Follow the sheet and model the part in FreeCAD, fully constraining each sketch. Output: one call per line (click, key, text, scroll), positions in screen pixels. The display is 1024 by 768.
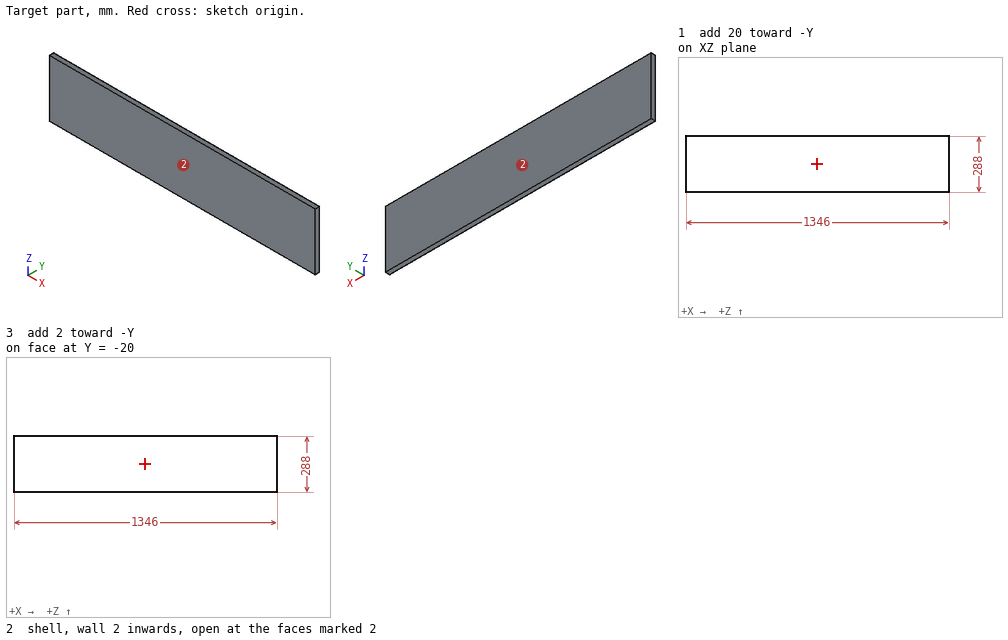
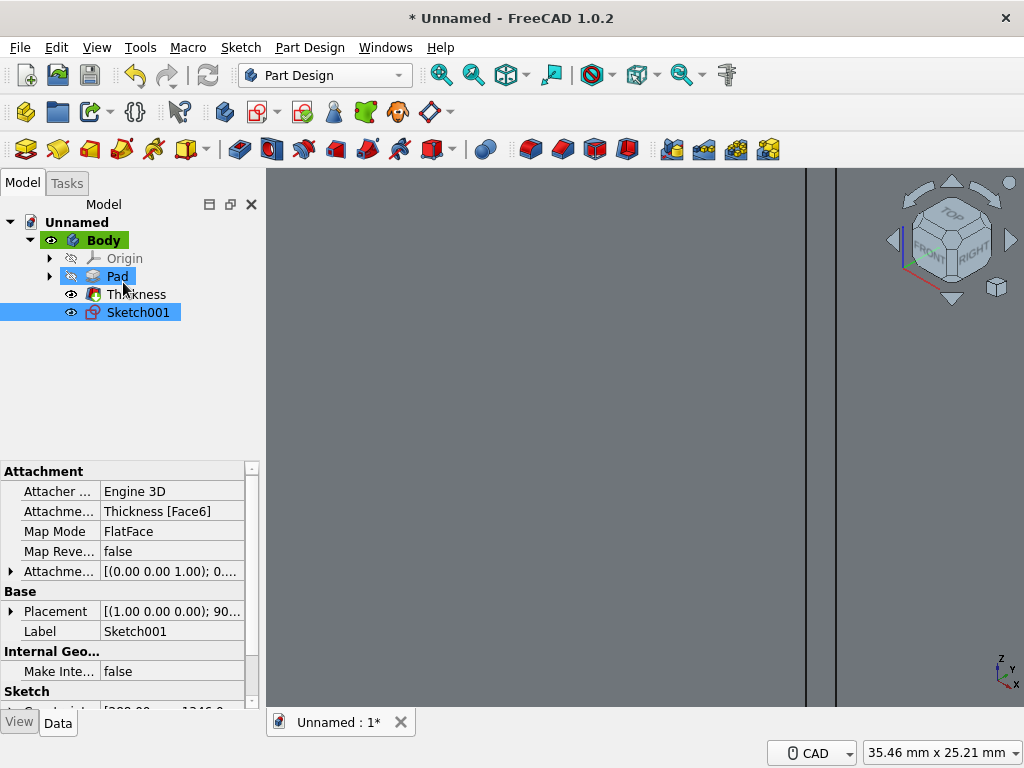
click(26, 150)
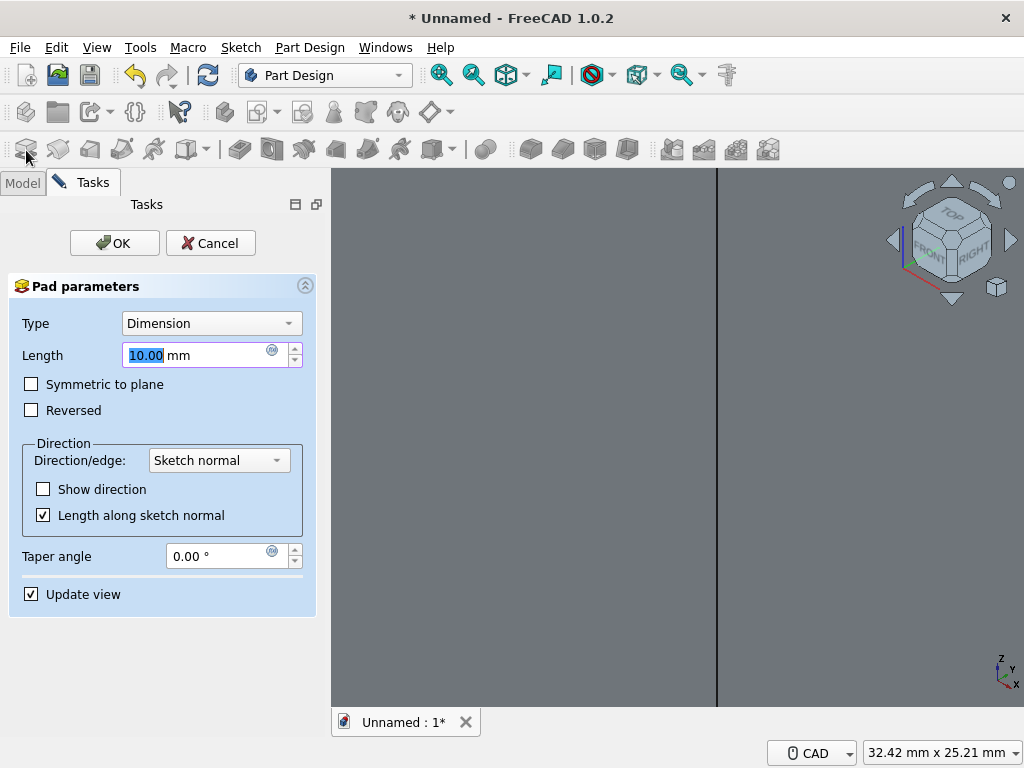
text(2)
key(Tab)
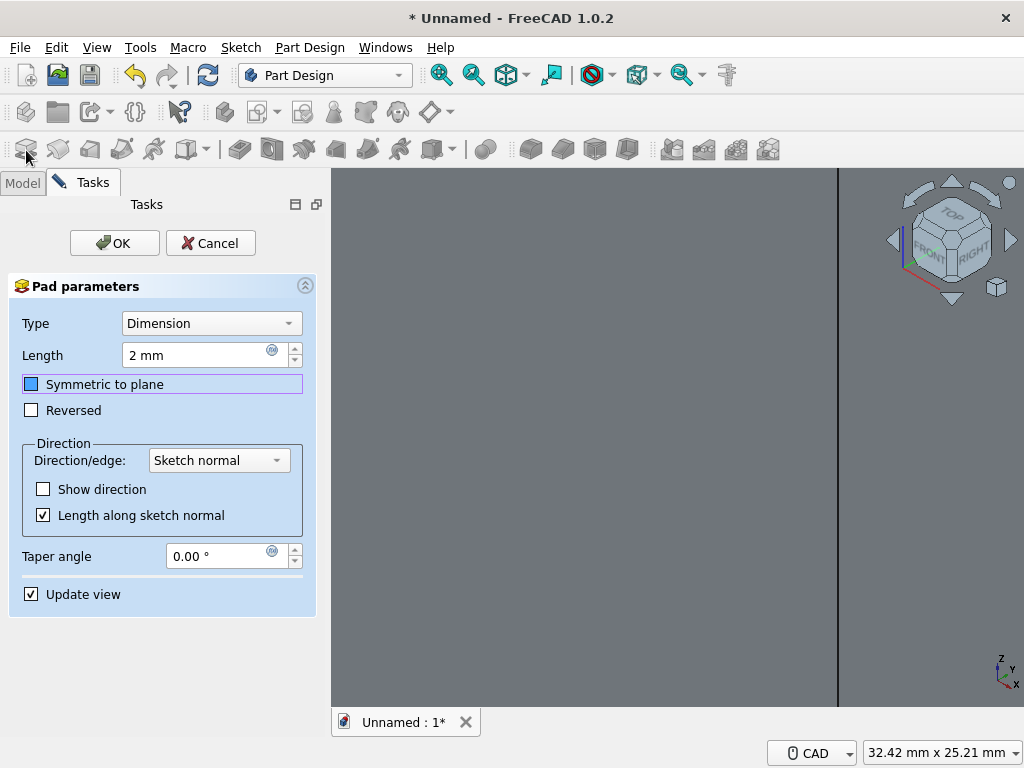
click(115, 243)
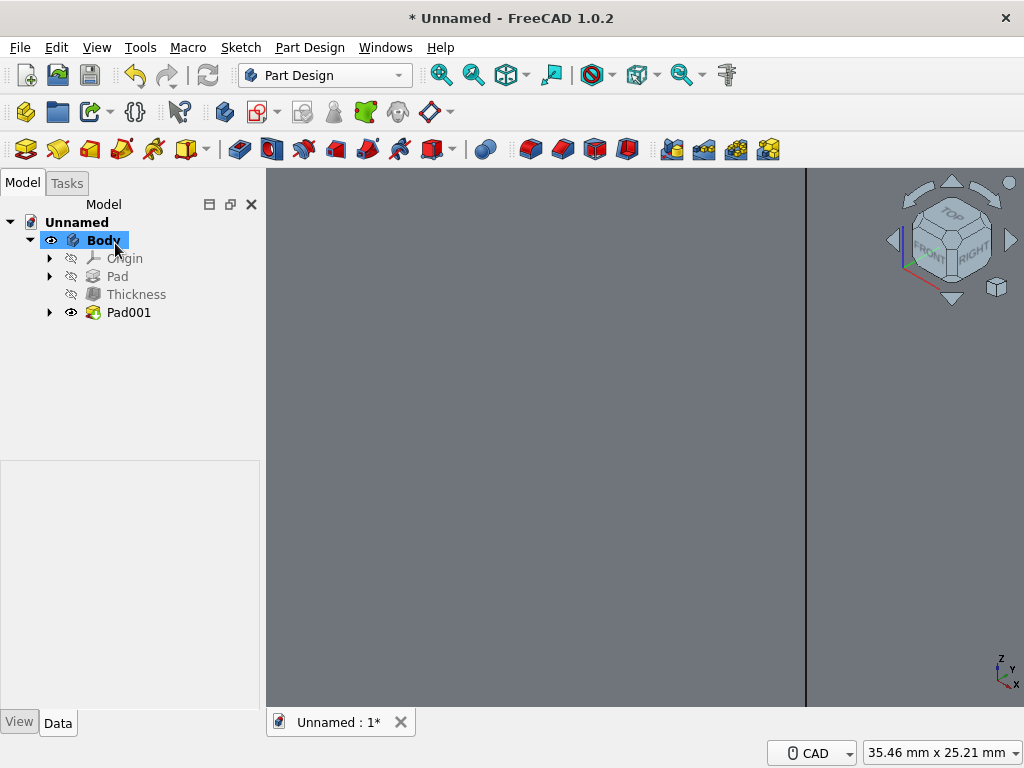
key(v)
key(f)